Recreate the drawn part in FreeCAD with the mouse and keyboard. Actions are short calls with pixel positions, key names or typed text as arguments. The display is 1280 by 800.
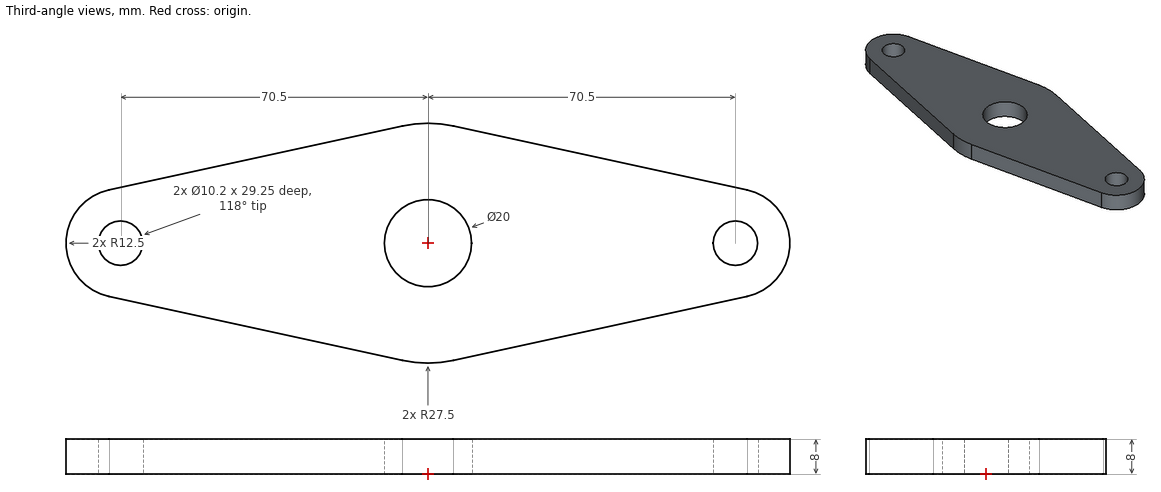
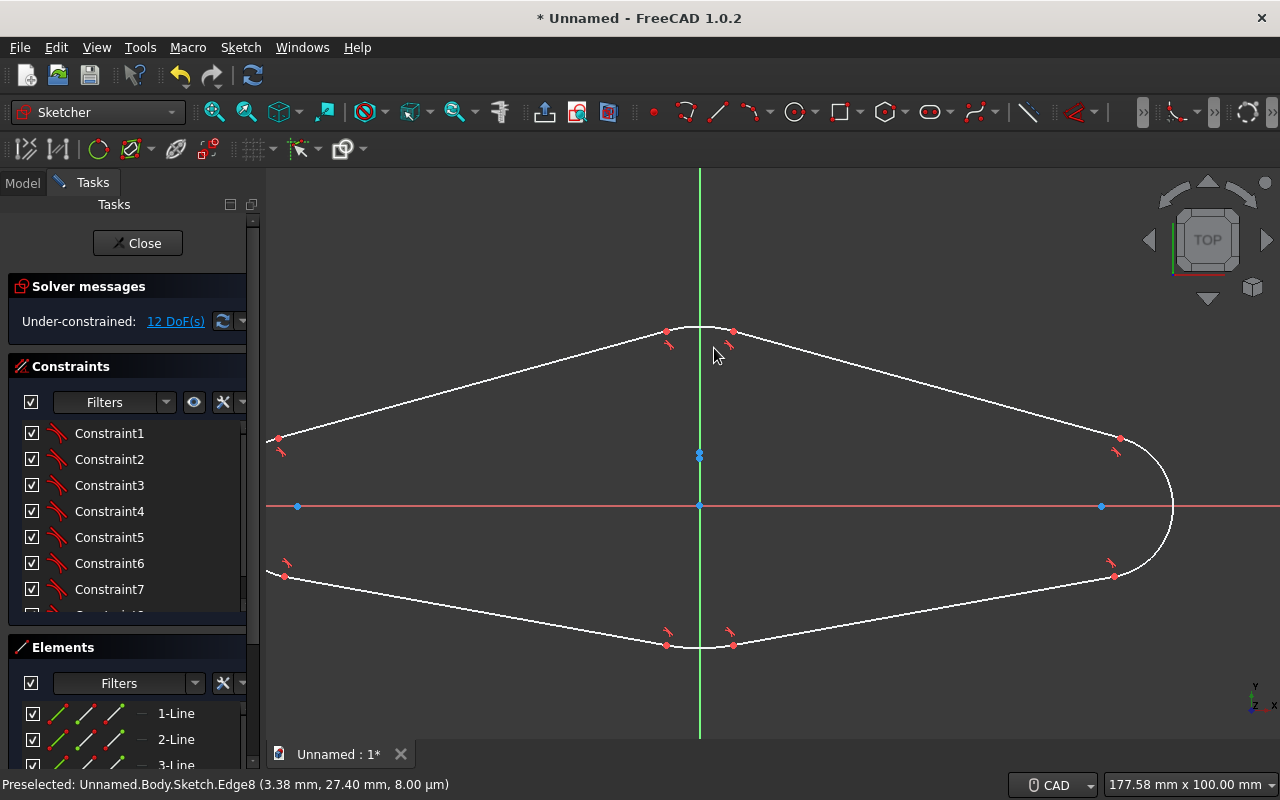
click(686, 648)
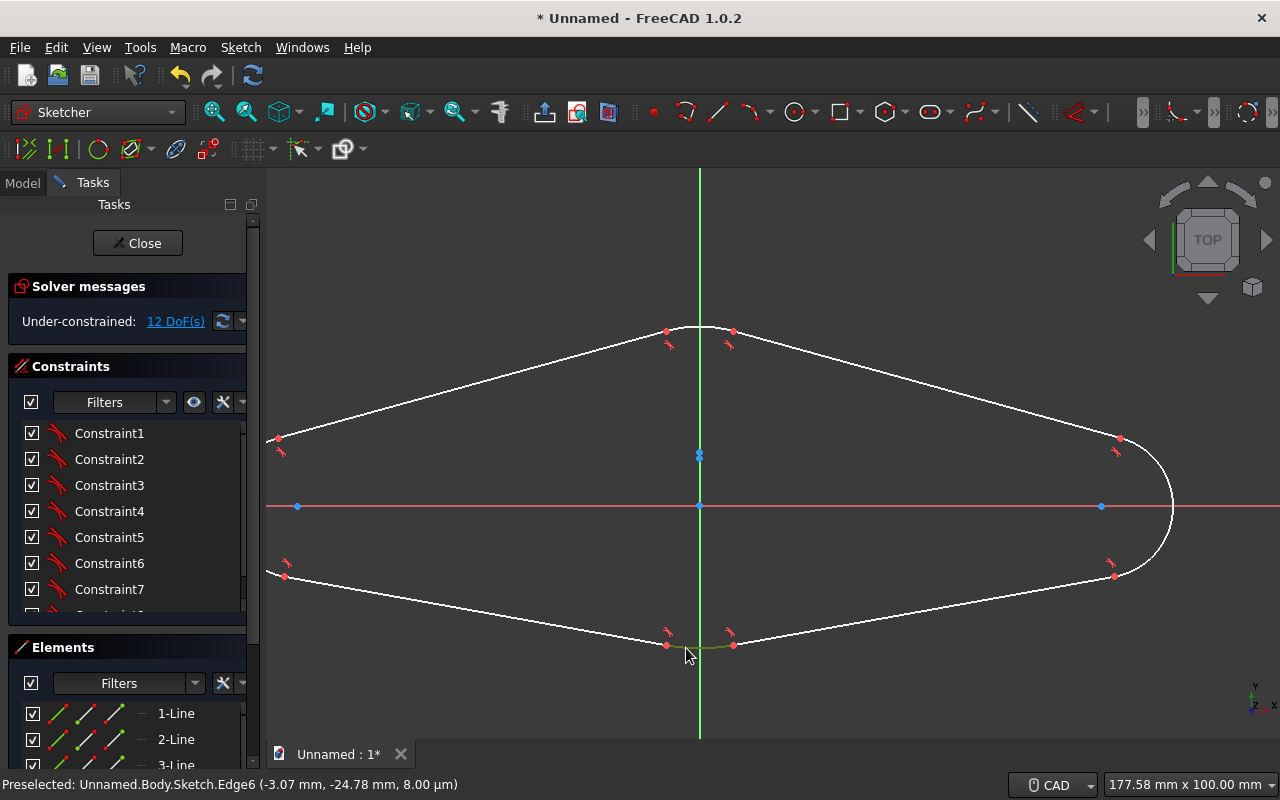
click(713, 327)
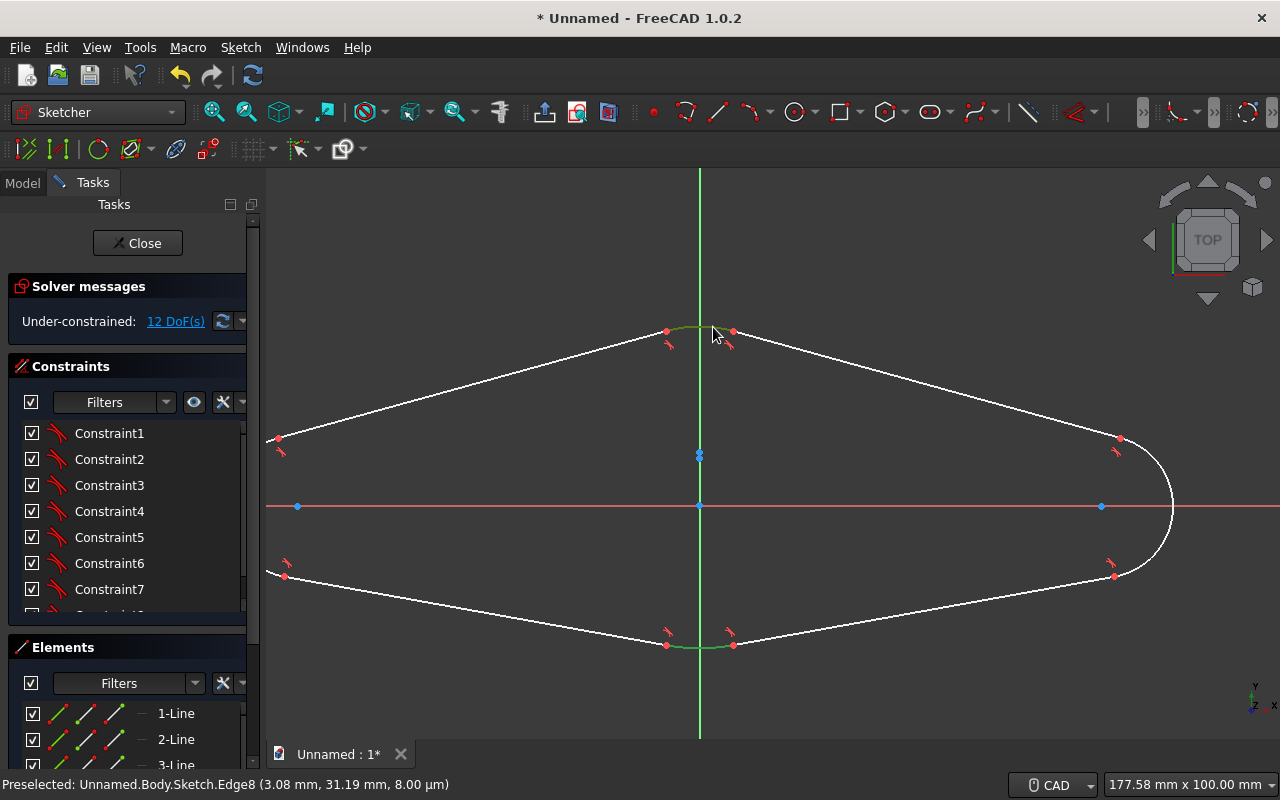
key(c)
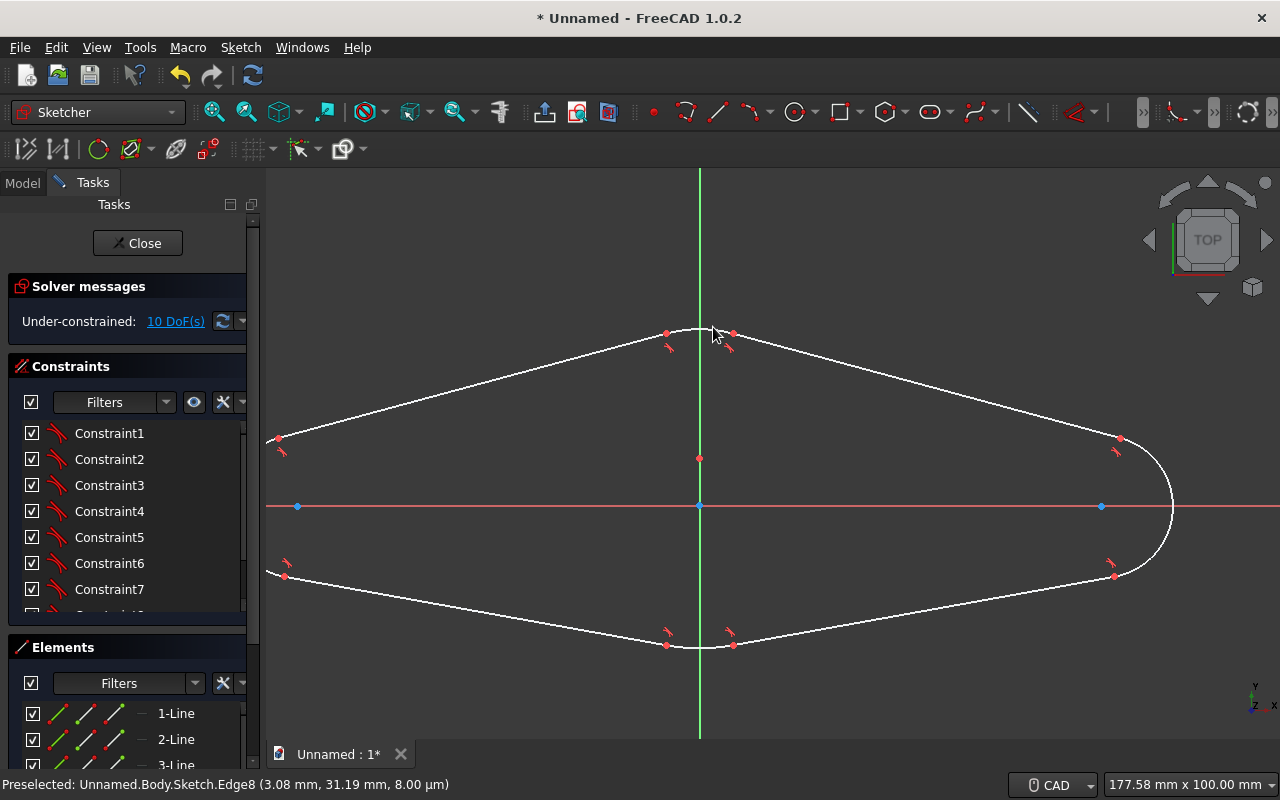
drag(690, 448, 710, 516)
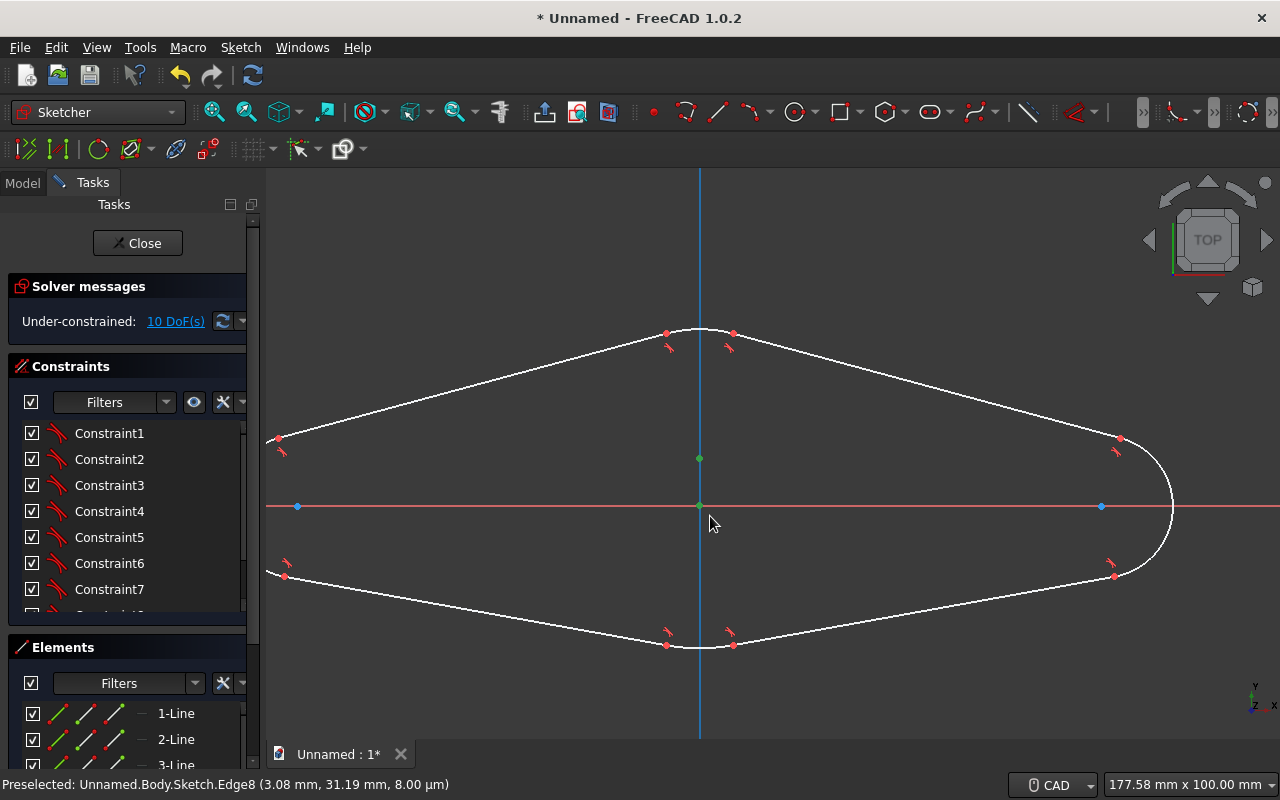
key(c)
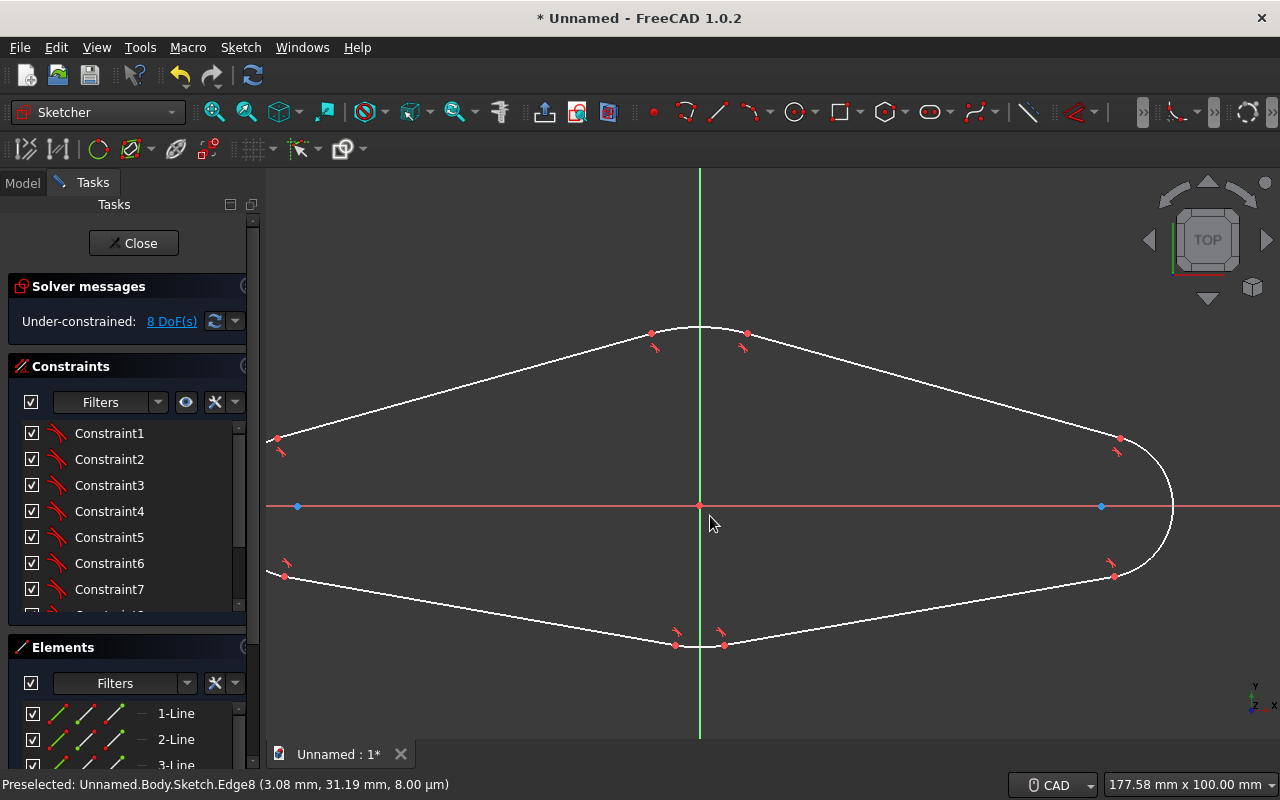
scroll(714, 347, down, 2)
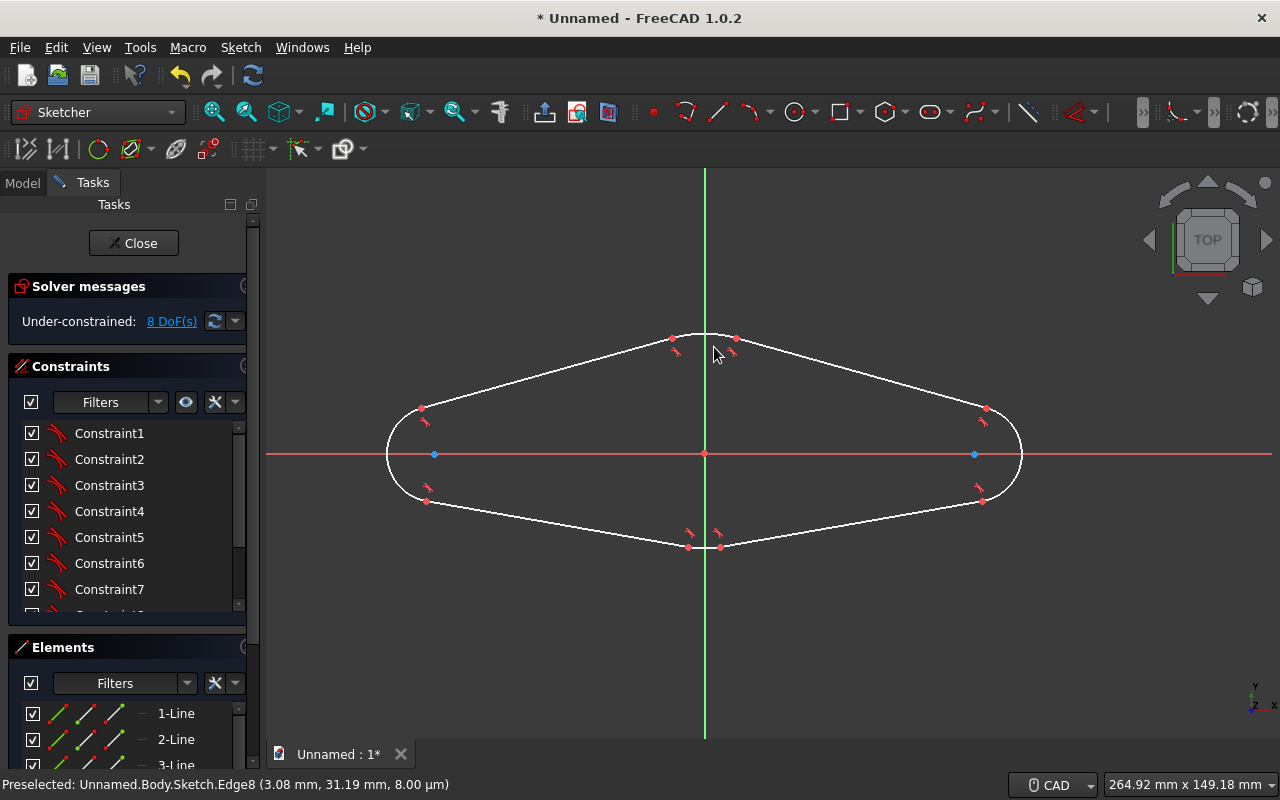
click(393, 432)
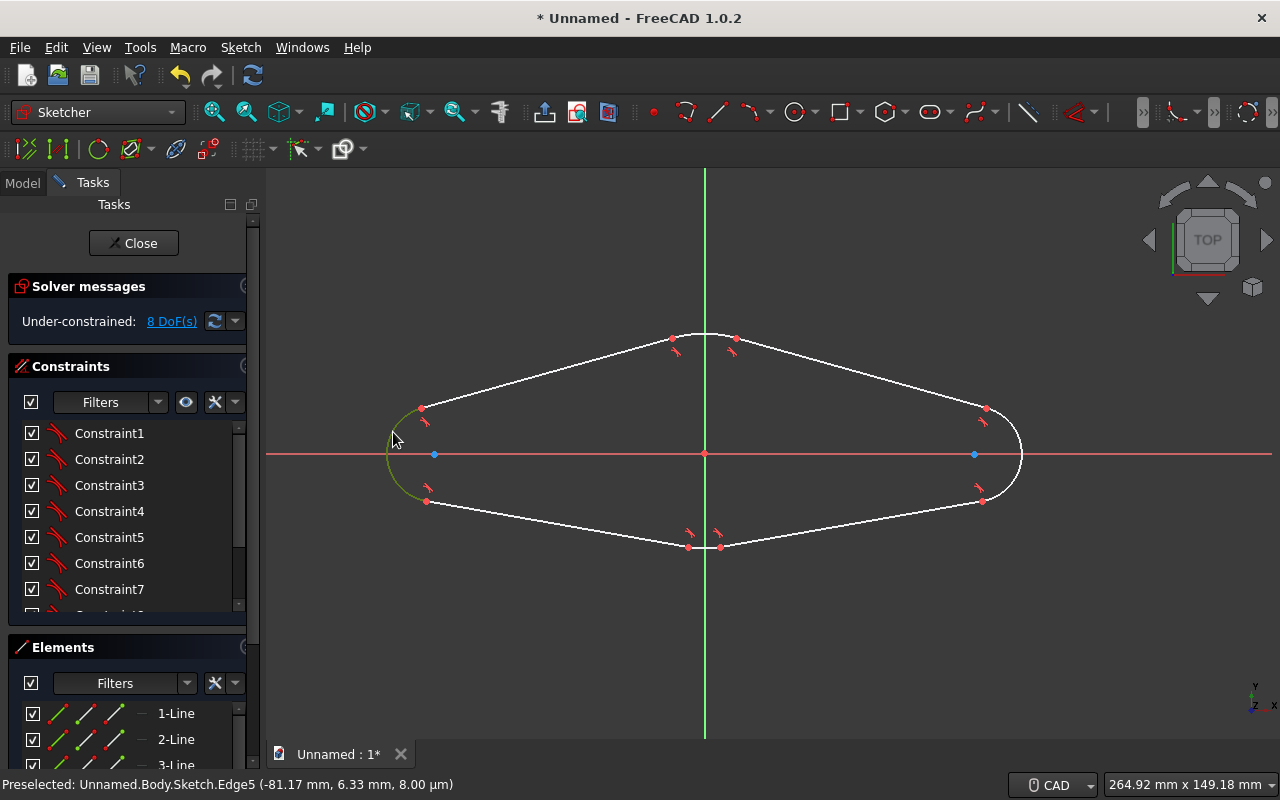
click(1014, 481)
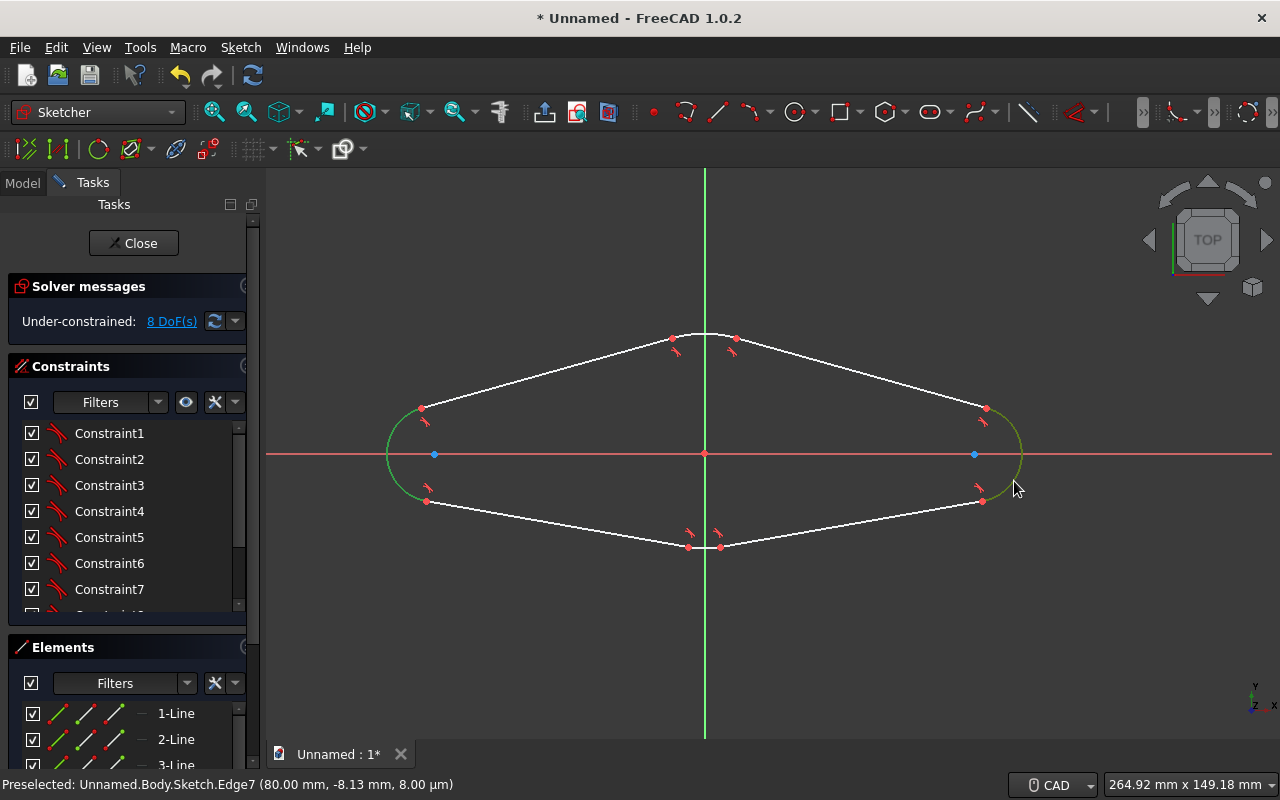
key(e)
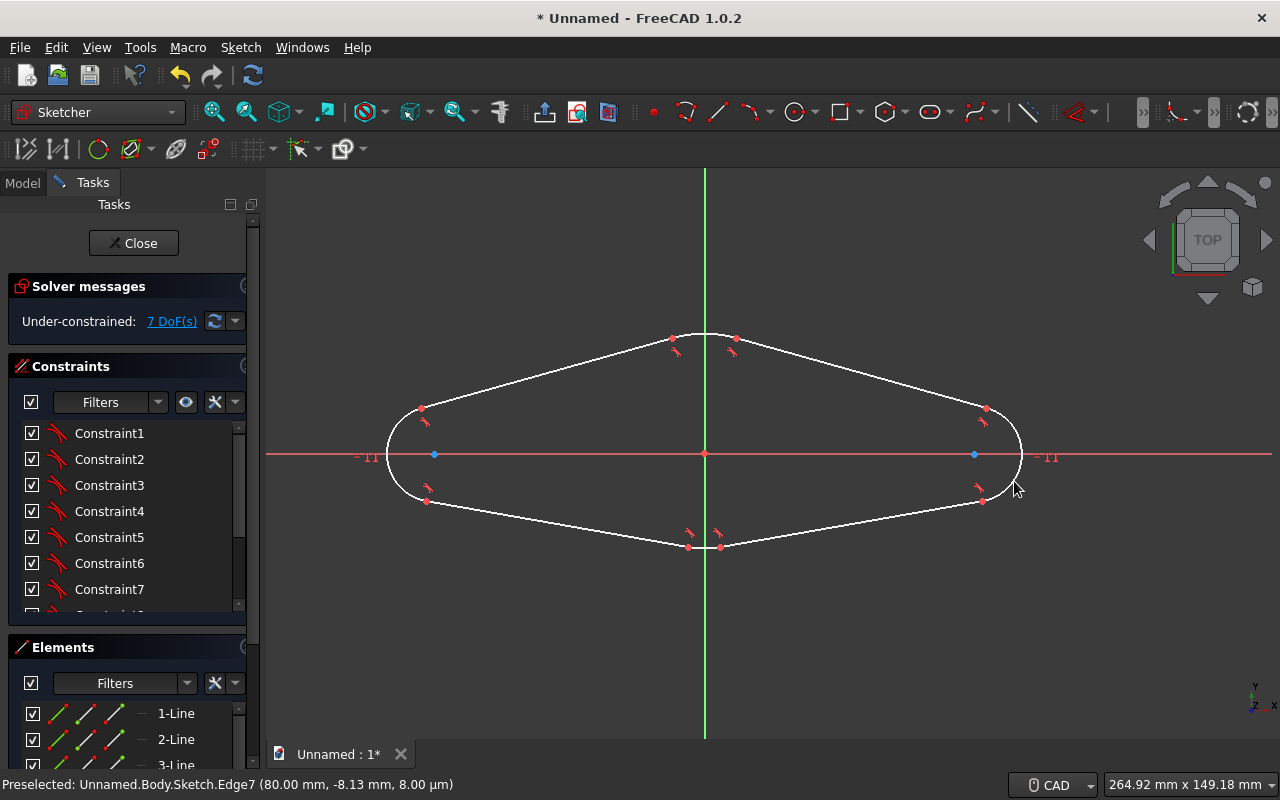
click(705, 548)